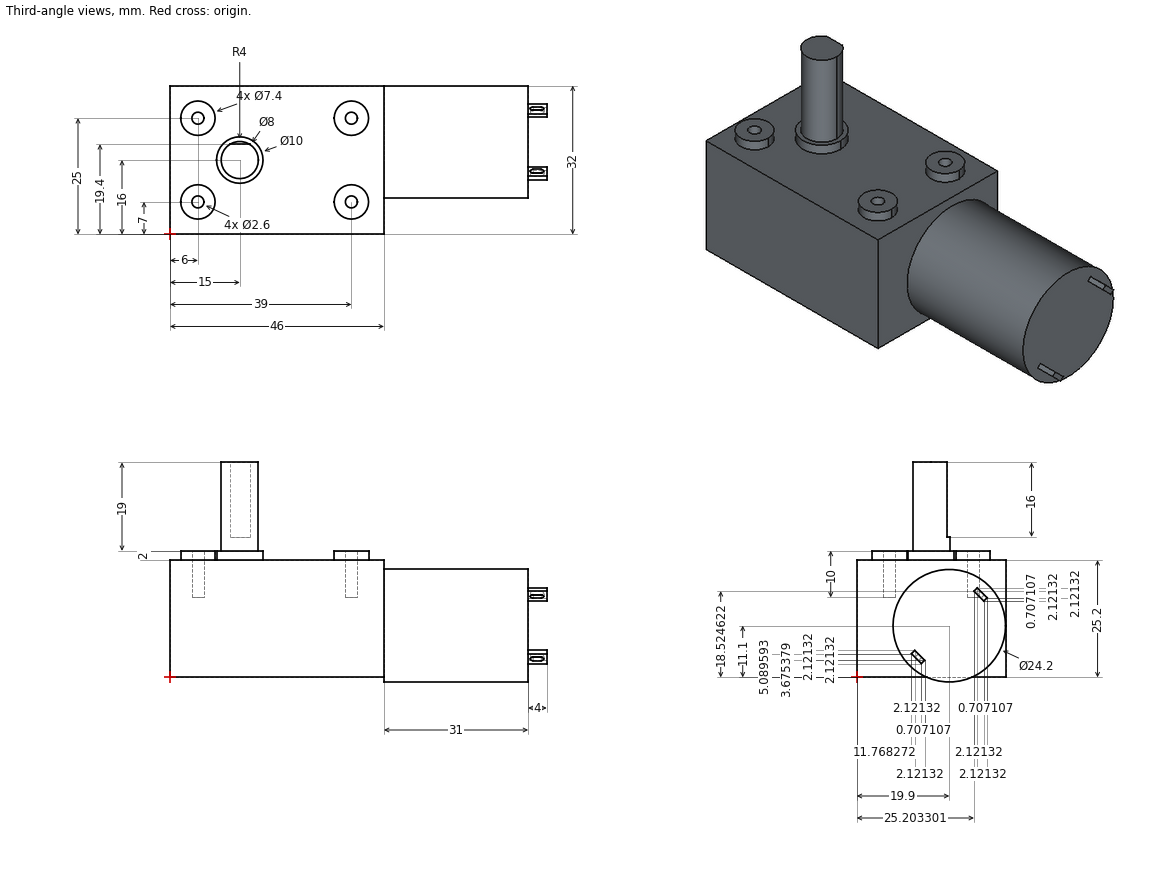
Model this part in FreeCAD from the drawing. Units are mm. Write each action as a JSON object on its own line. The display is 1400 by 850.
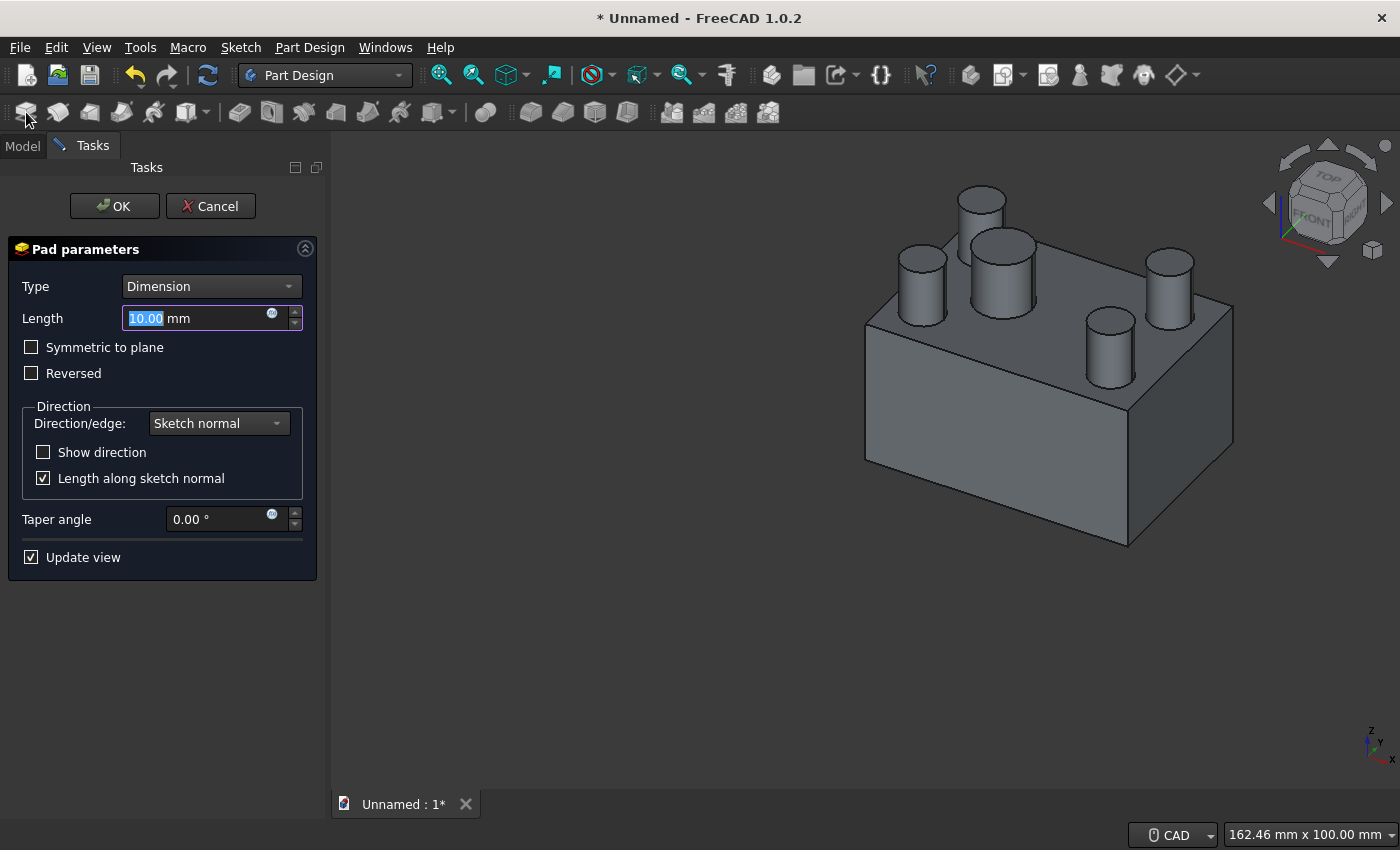
{"action": "type", "text": "2"}
{"action": "key", "text": "Tab"}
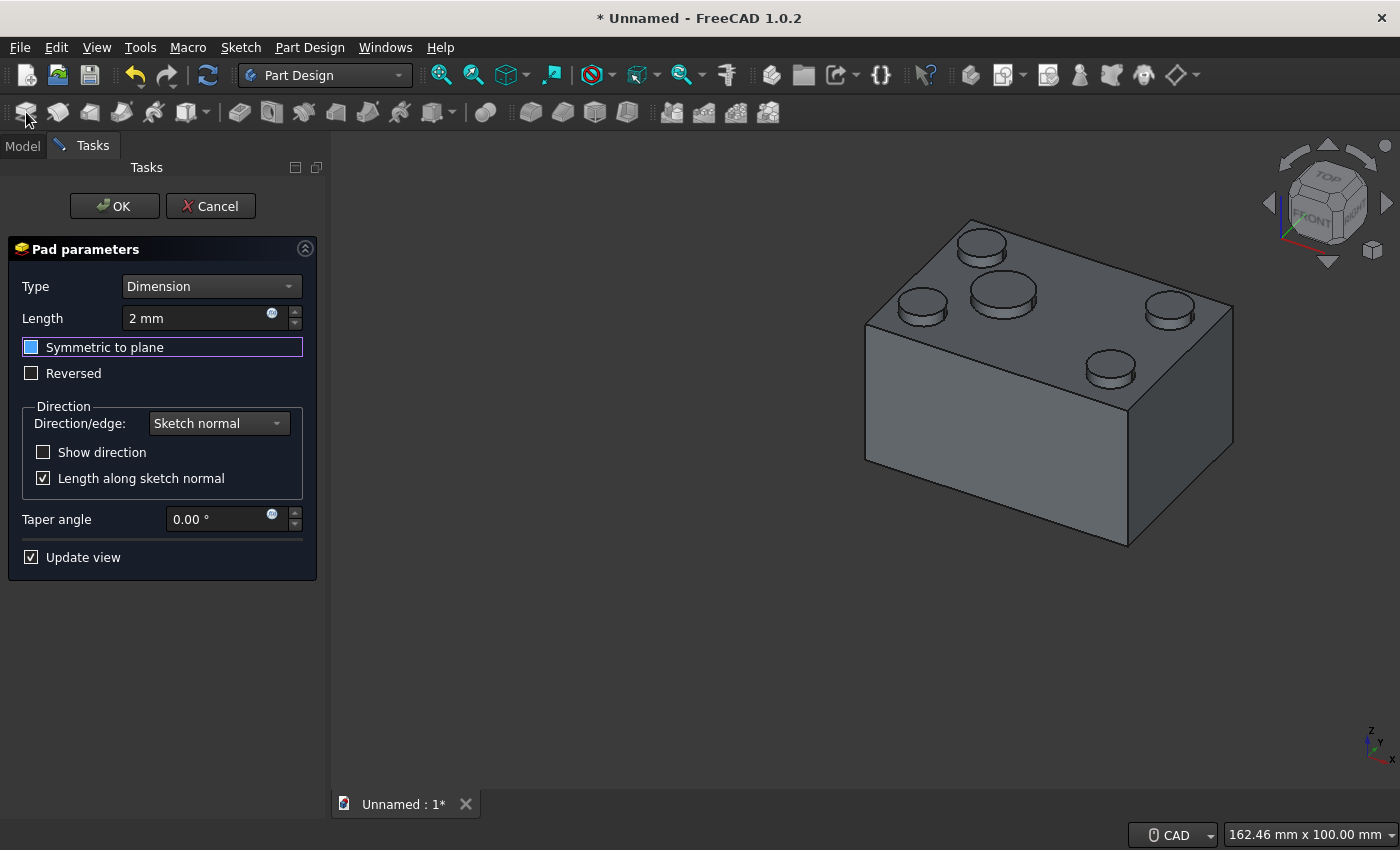
{"action": "left_click", "coordinate": [115, 206]}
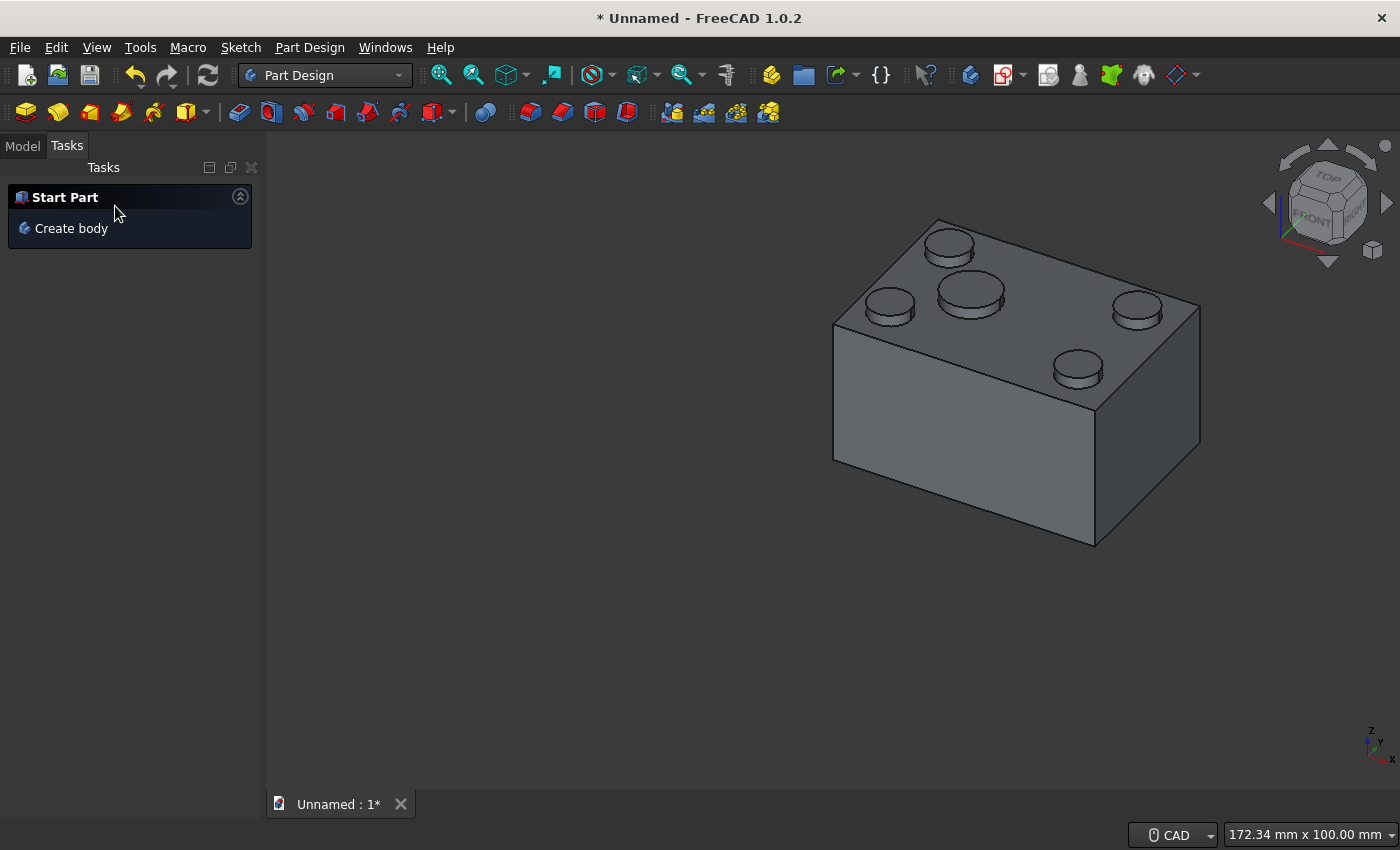
{"action": "left_click", "coordinate": [971, 288]}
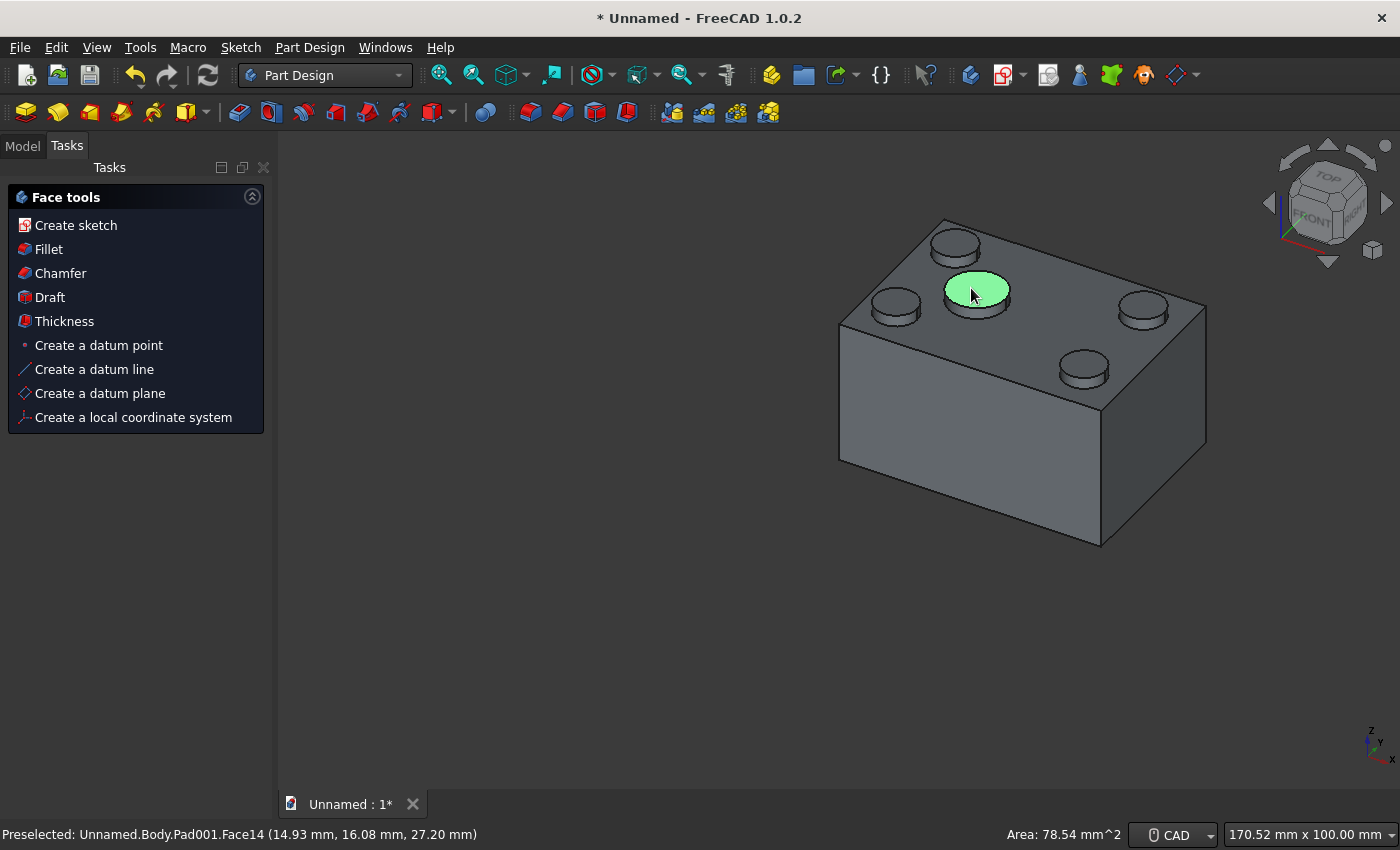
{"action": "left_click", "coordinate": [1004, 76]}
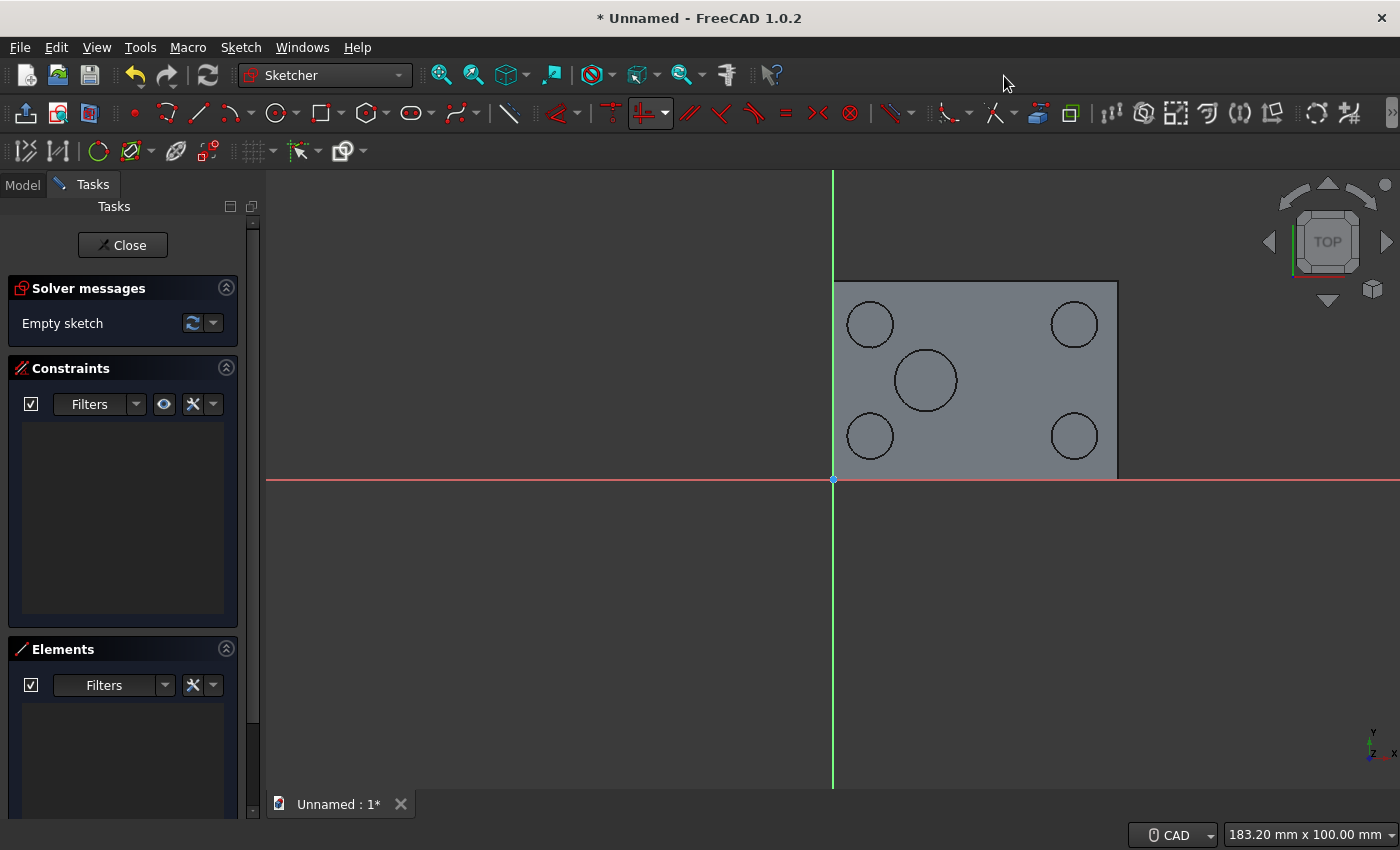
{"action": "scroll", "coordinate": [1115, 332], "scroll_direction": "up", "scroll_amount": 4}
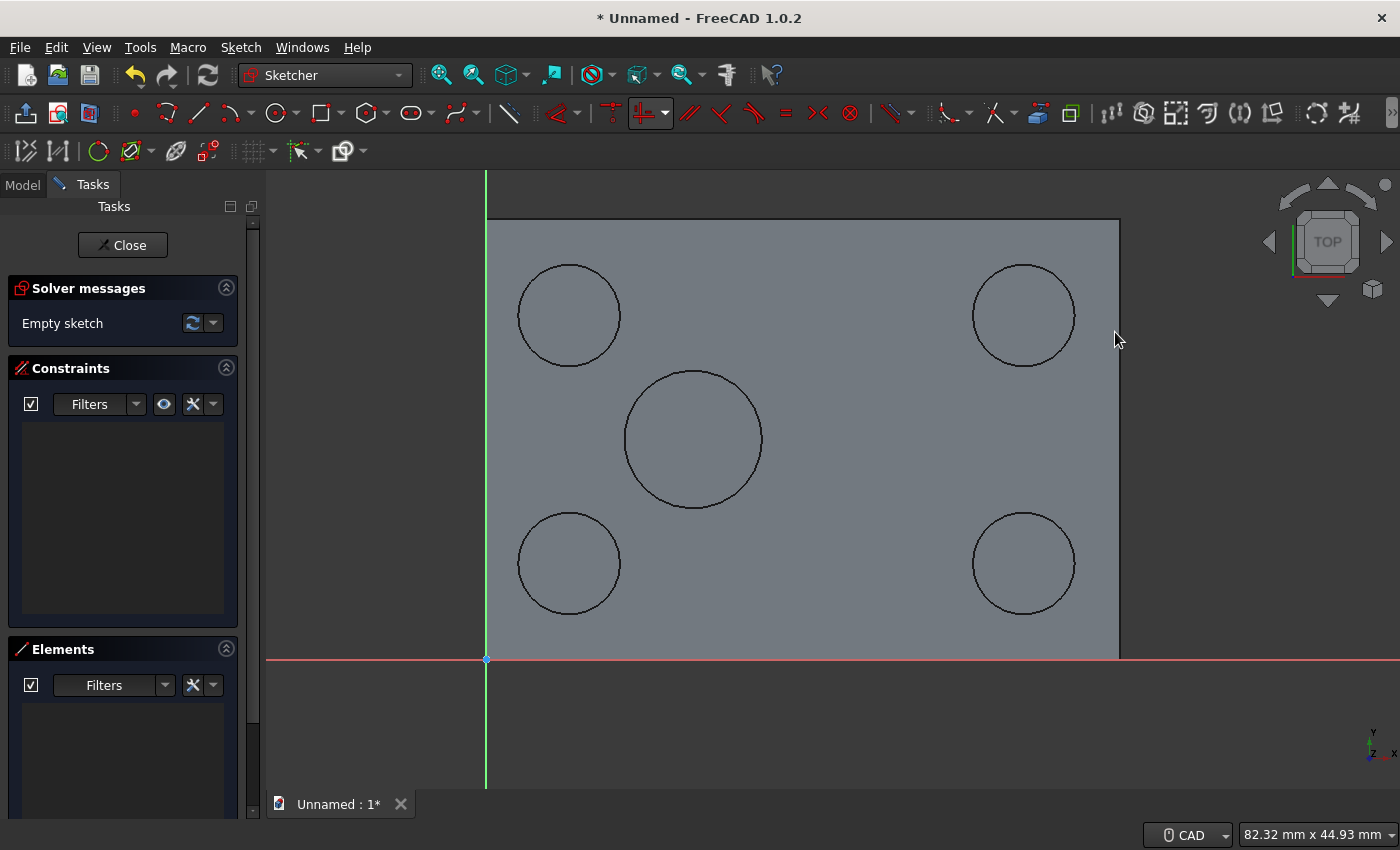
{"action": "left_click", "coordinate": [276, 114]}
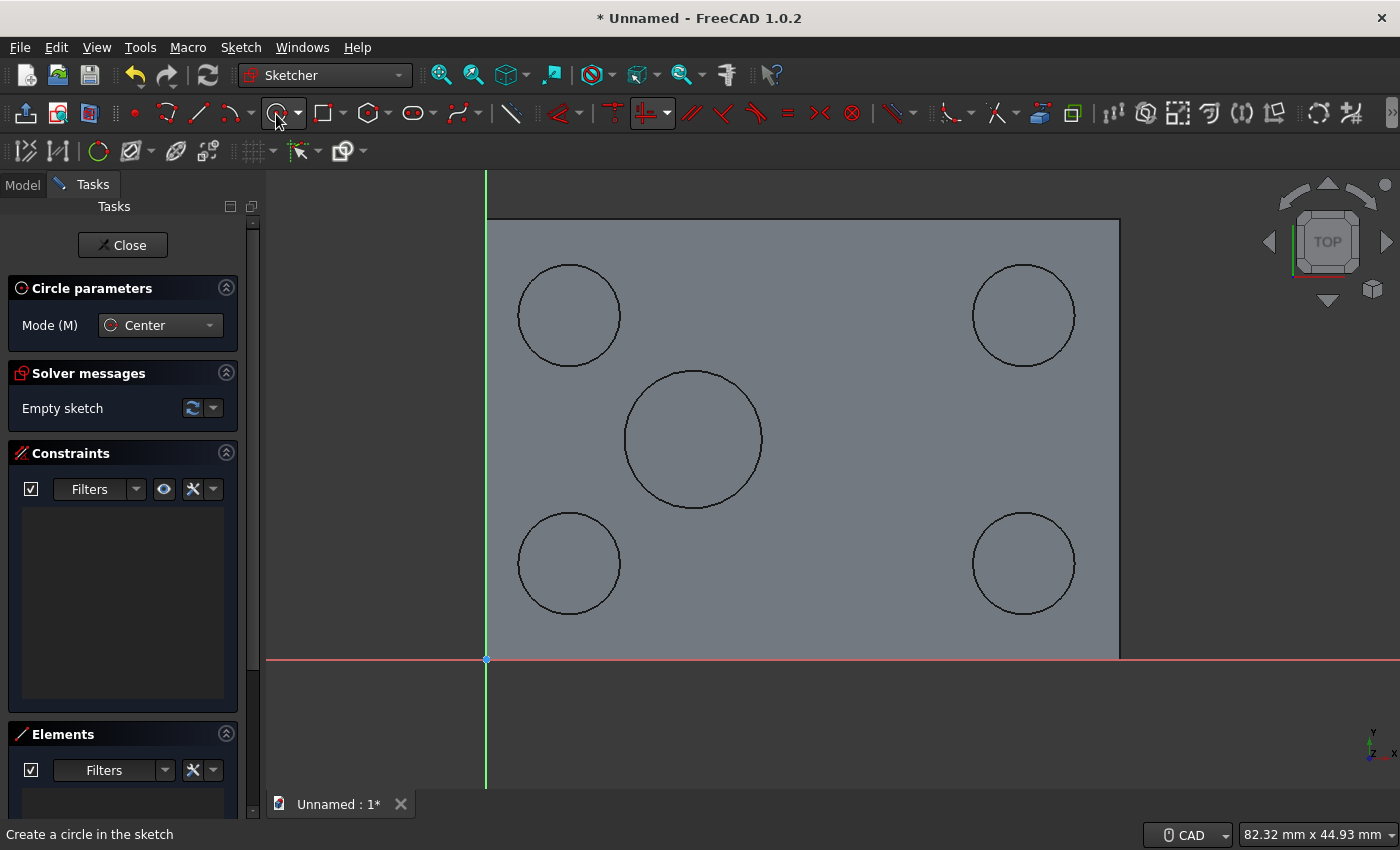
{"action": "scroll", "coordinate": [569, 564], "scroll_direction": "up", "scroll_amount": 2}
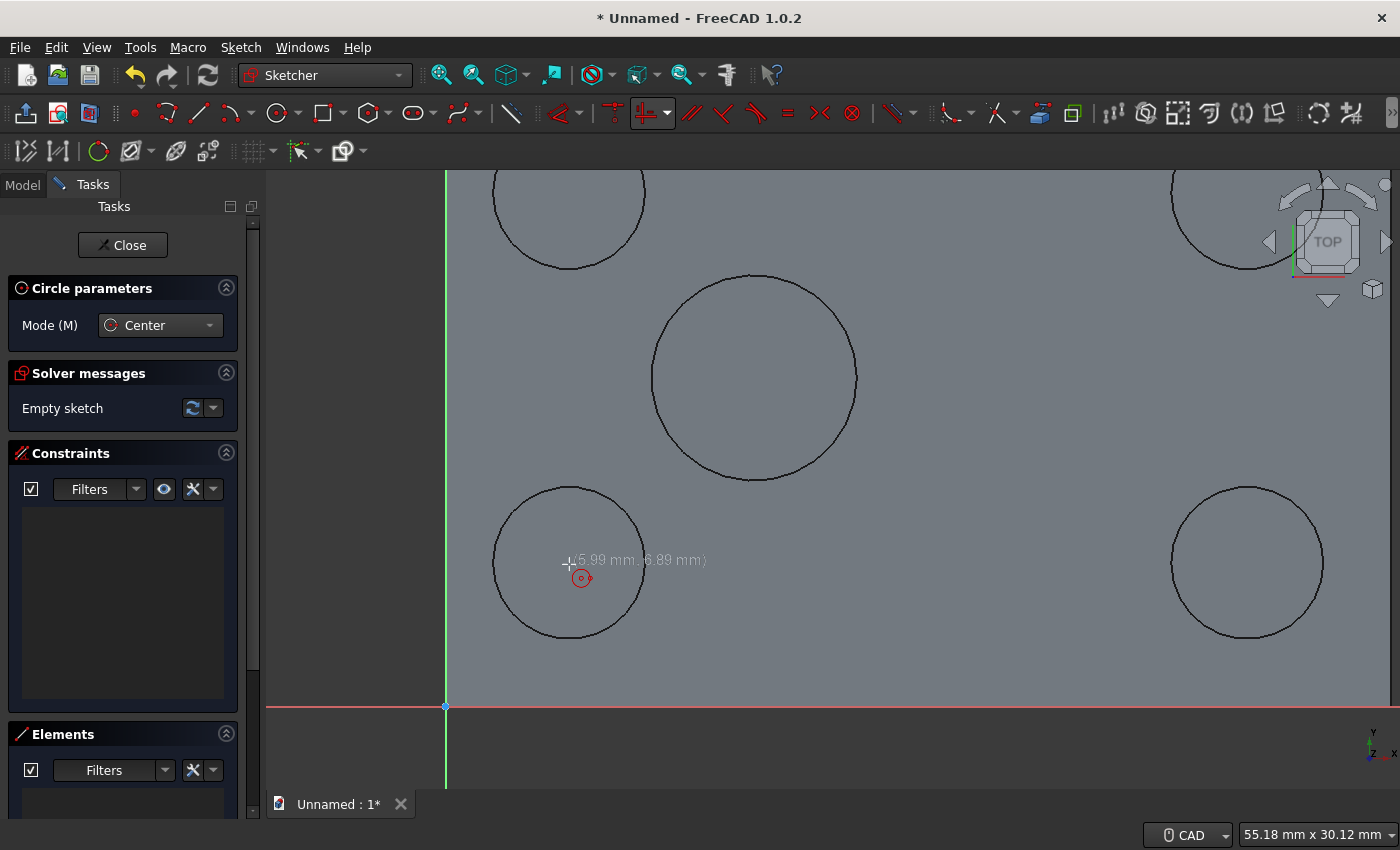
{"action": "left_click", "coordinate": [569, 563]}
{"action": "mouse_move", "coordinate": [588, 544]}